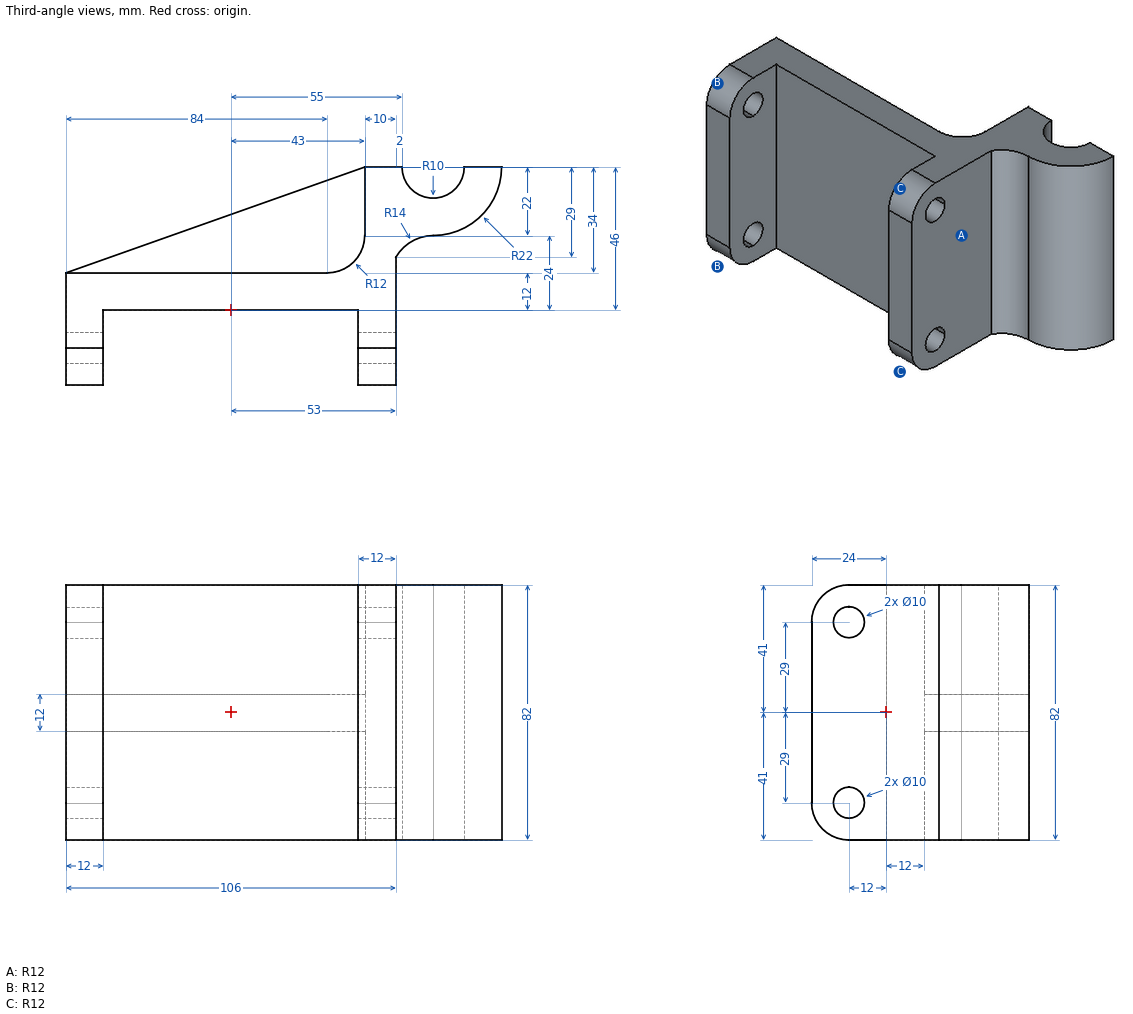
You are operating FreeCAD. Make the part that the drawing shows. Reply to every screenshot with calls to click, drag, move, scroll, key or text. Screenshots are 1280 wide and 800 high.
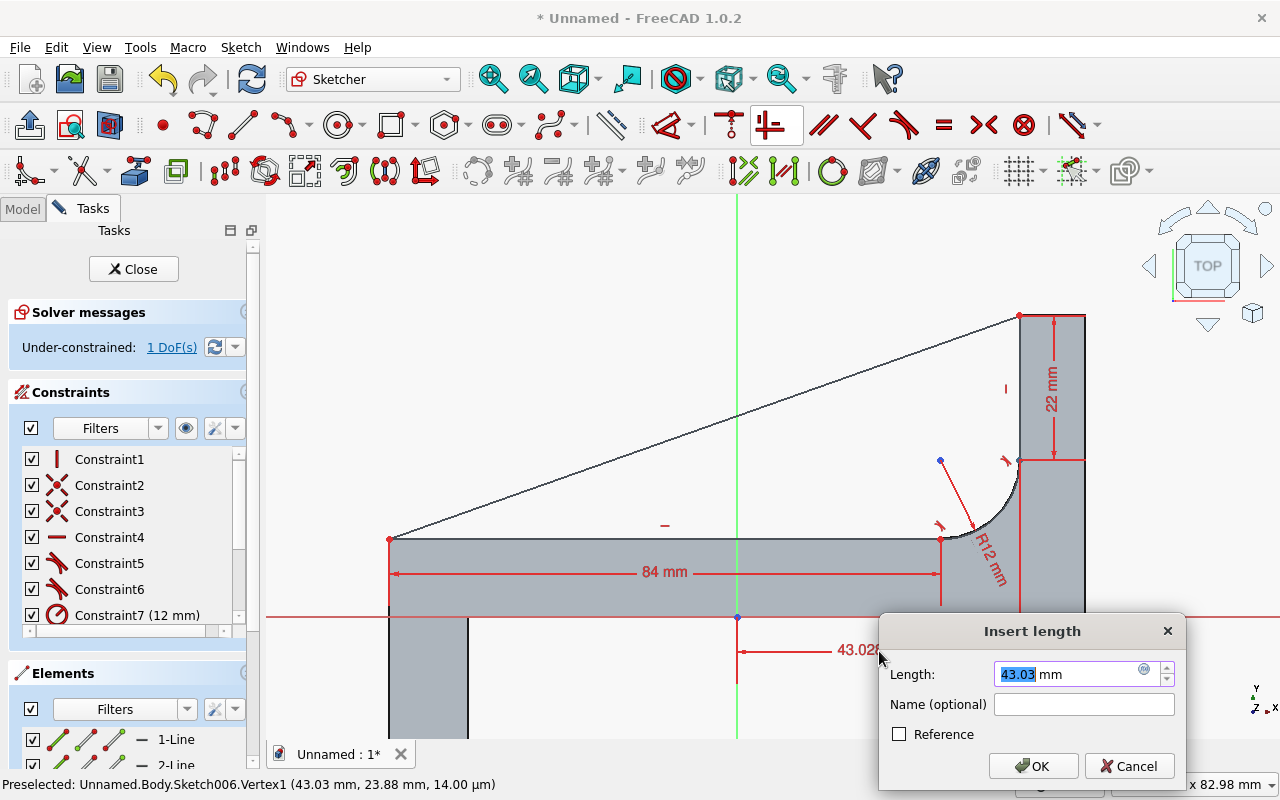
text(43)
key(Return)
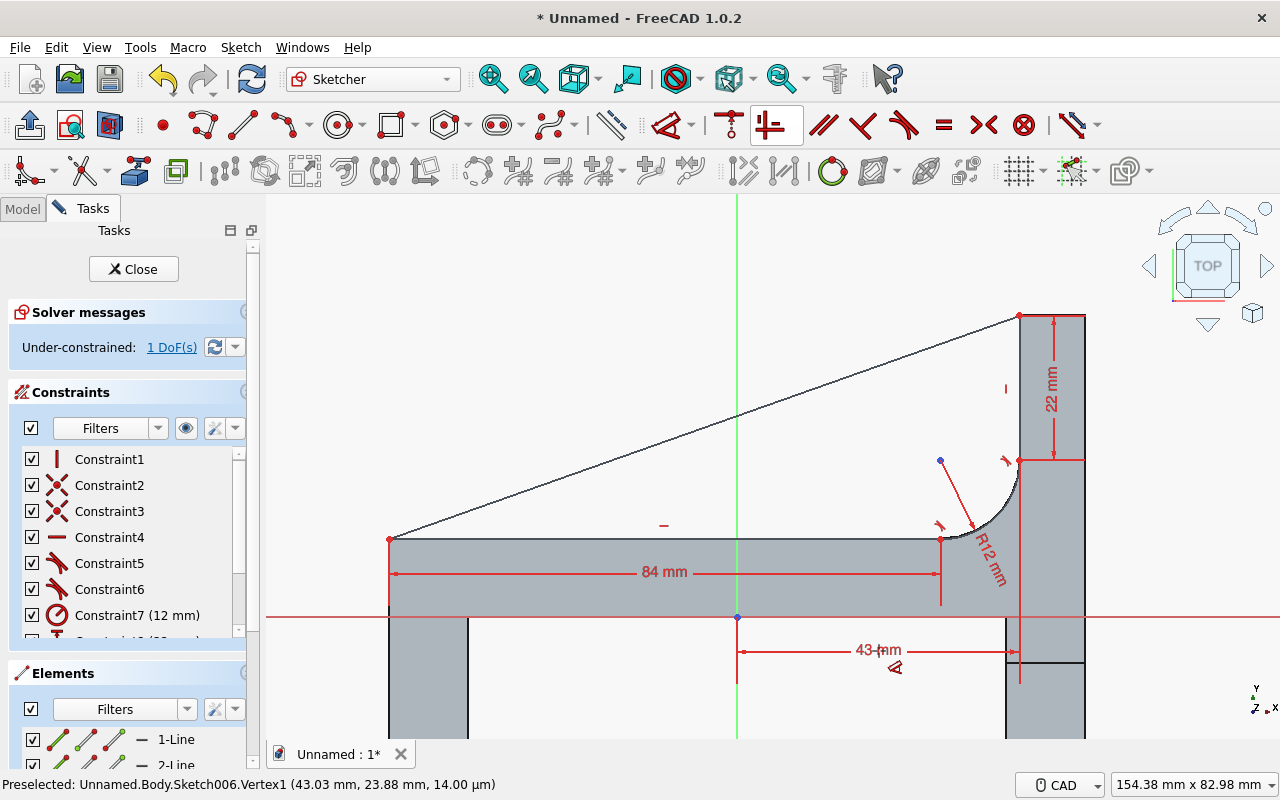
click(1020, 460)
click(1054, 539)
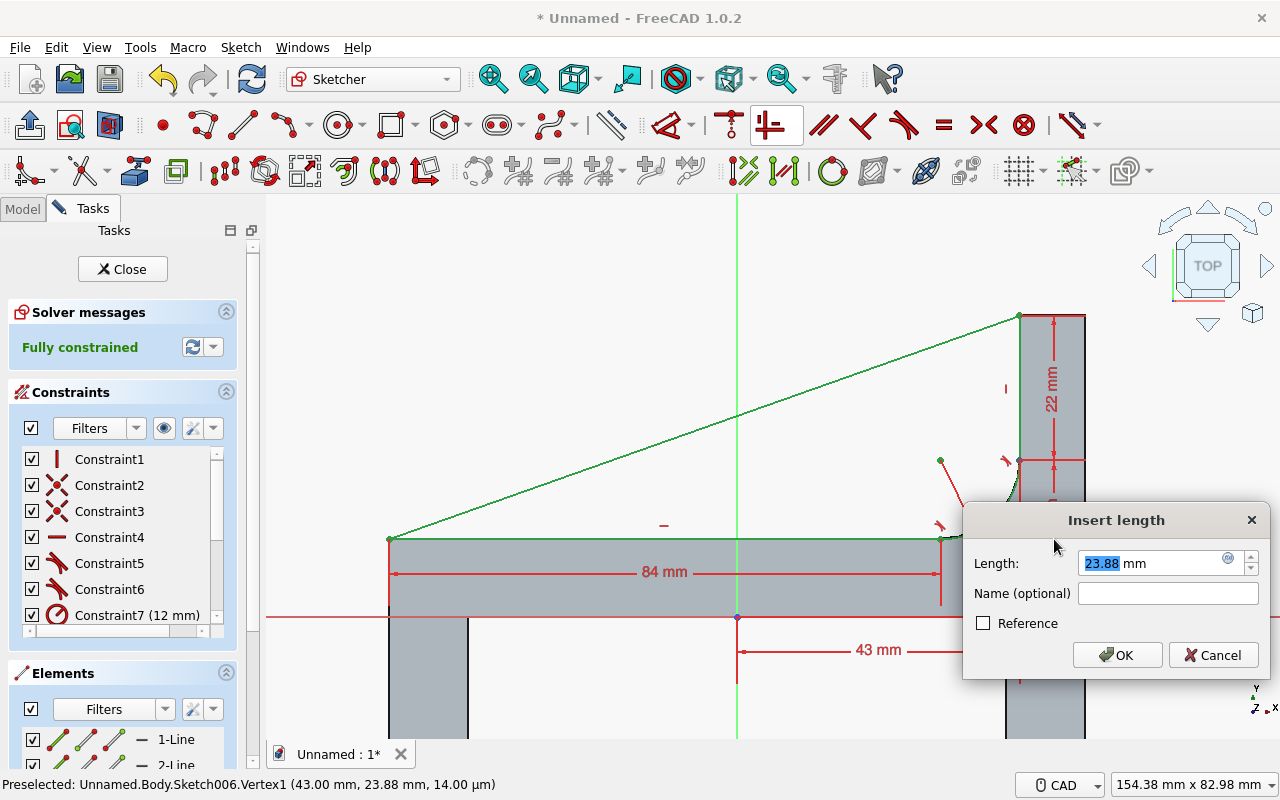
text(24)
key(Return)
key(Escape)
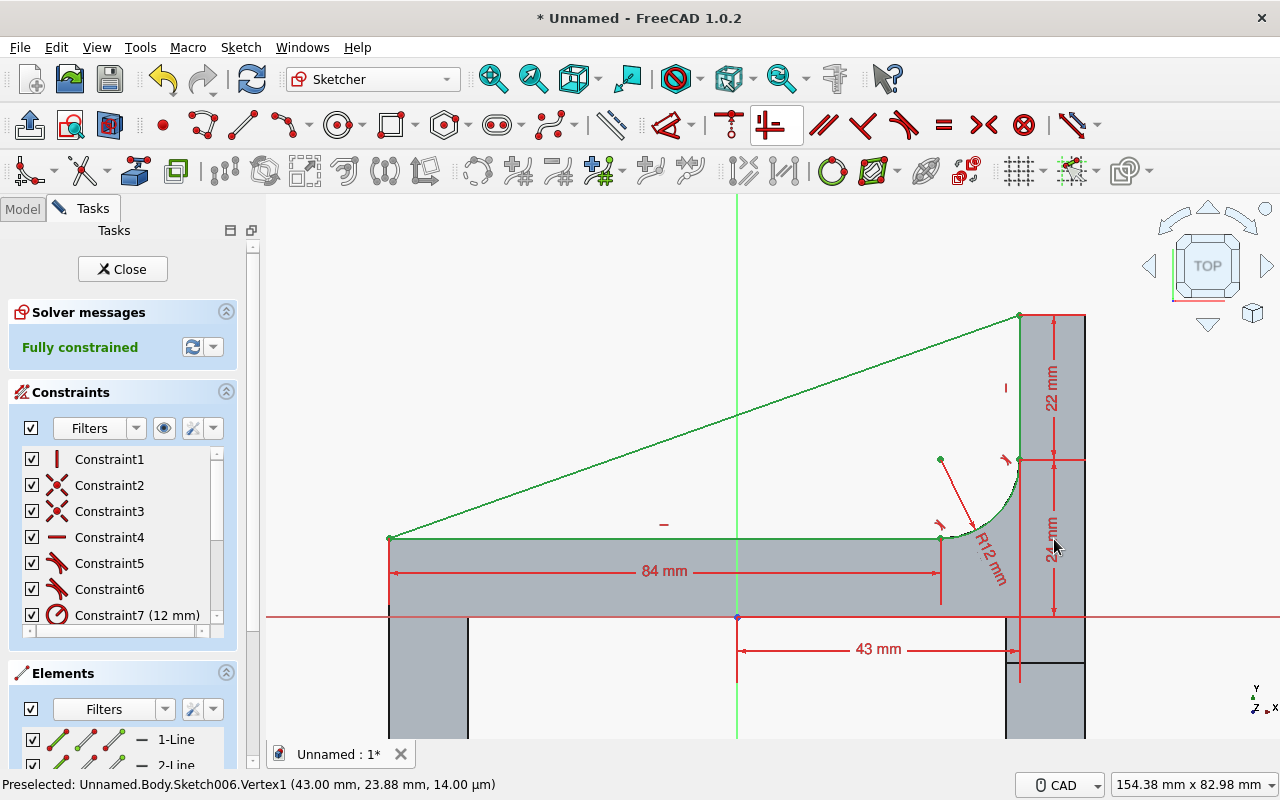
click(123, 269)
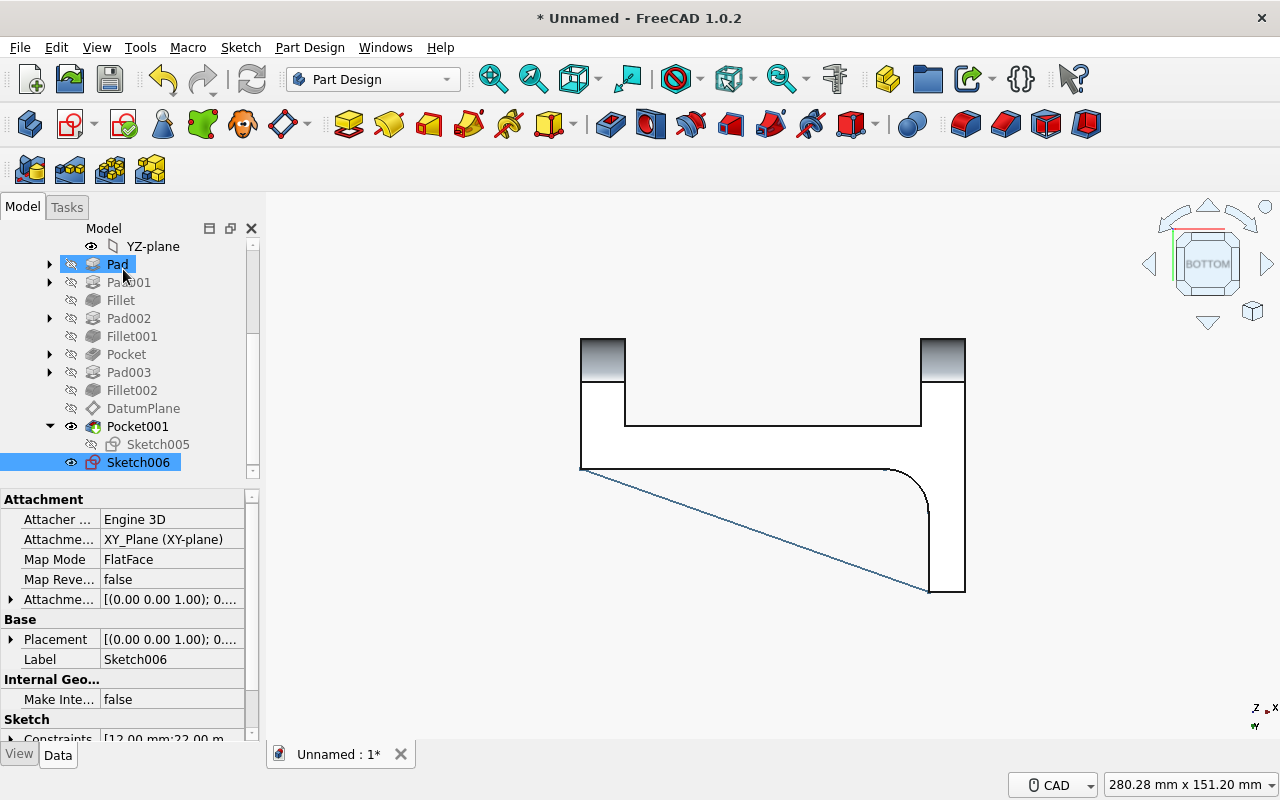
click(350, 124)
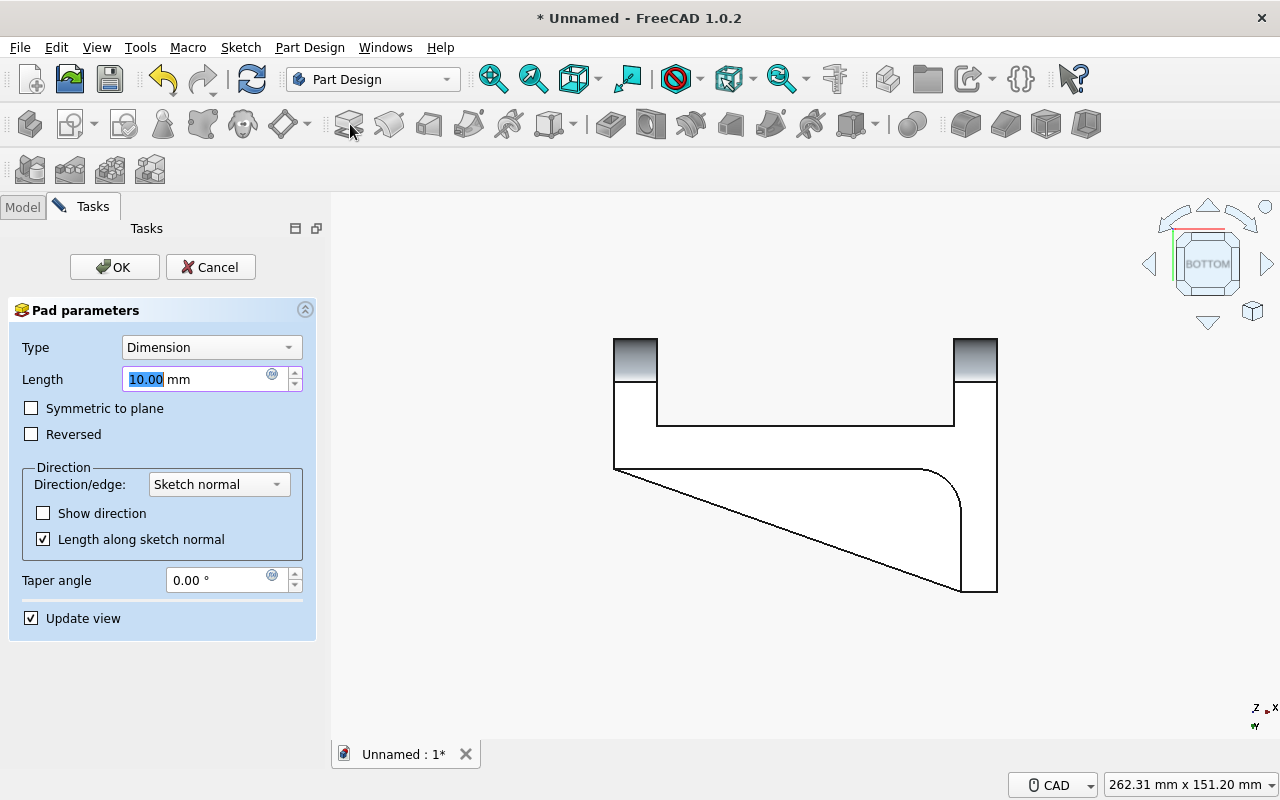
text(12)
key(Tab)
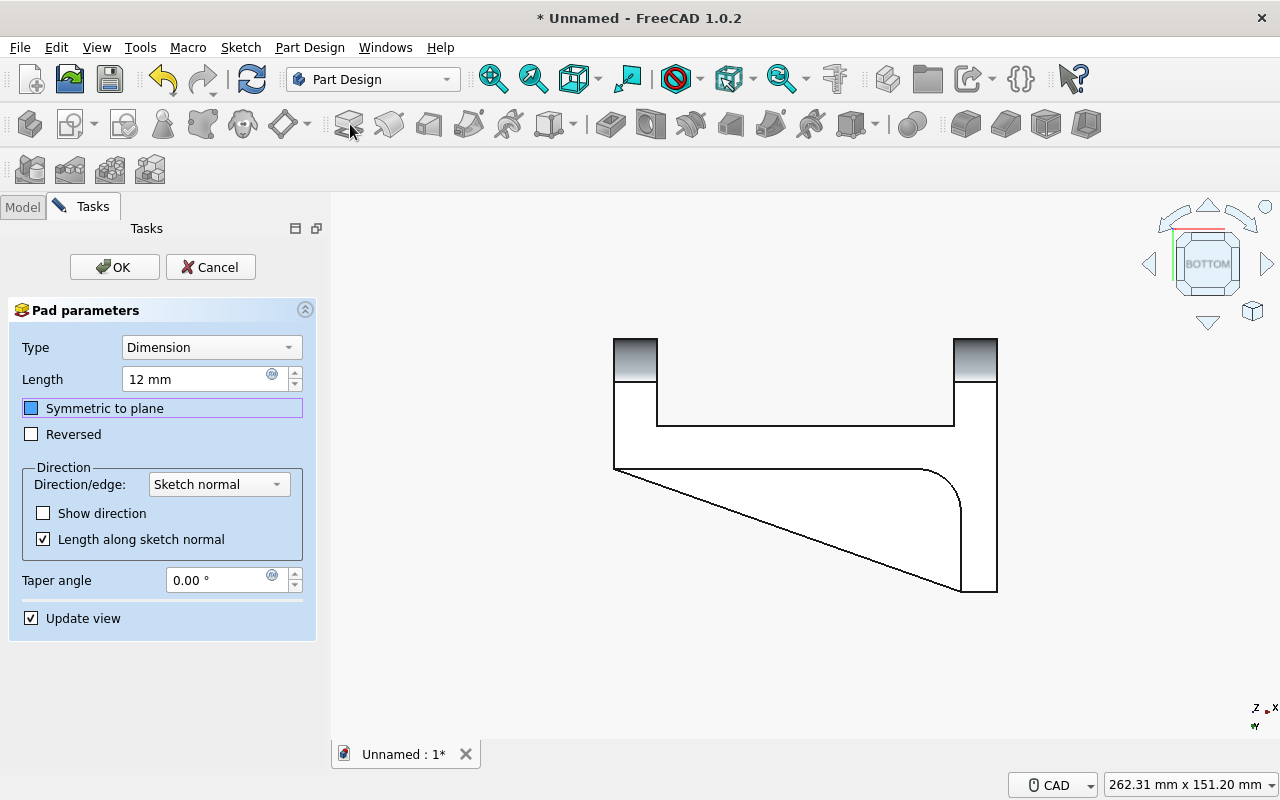
click(30, 408)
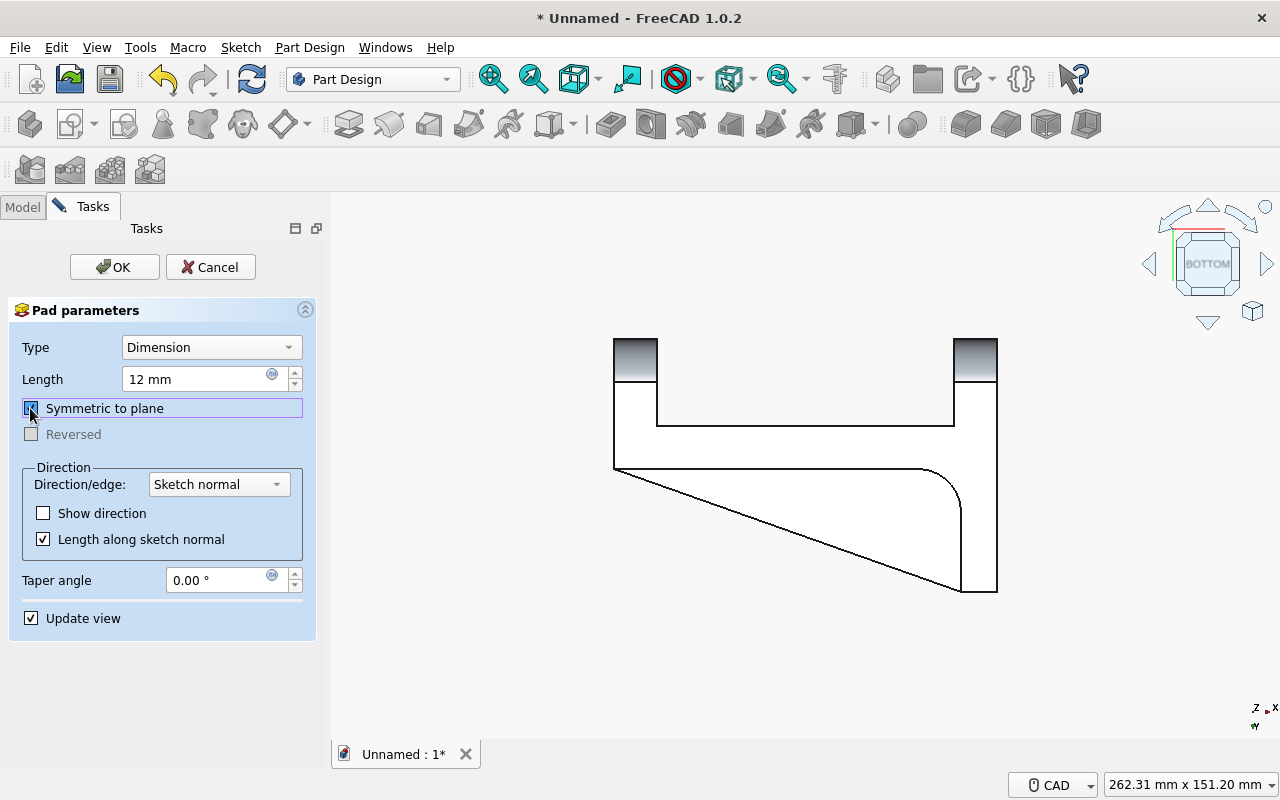
click(115, 267)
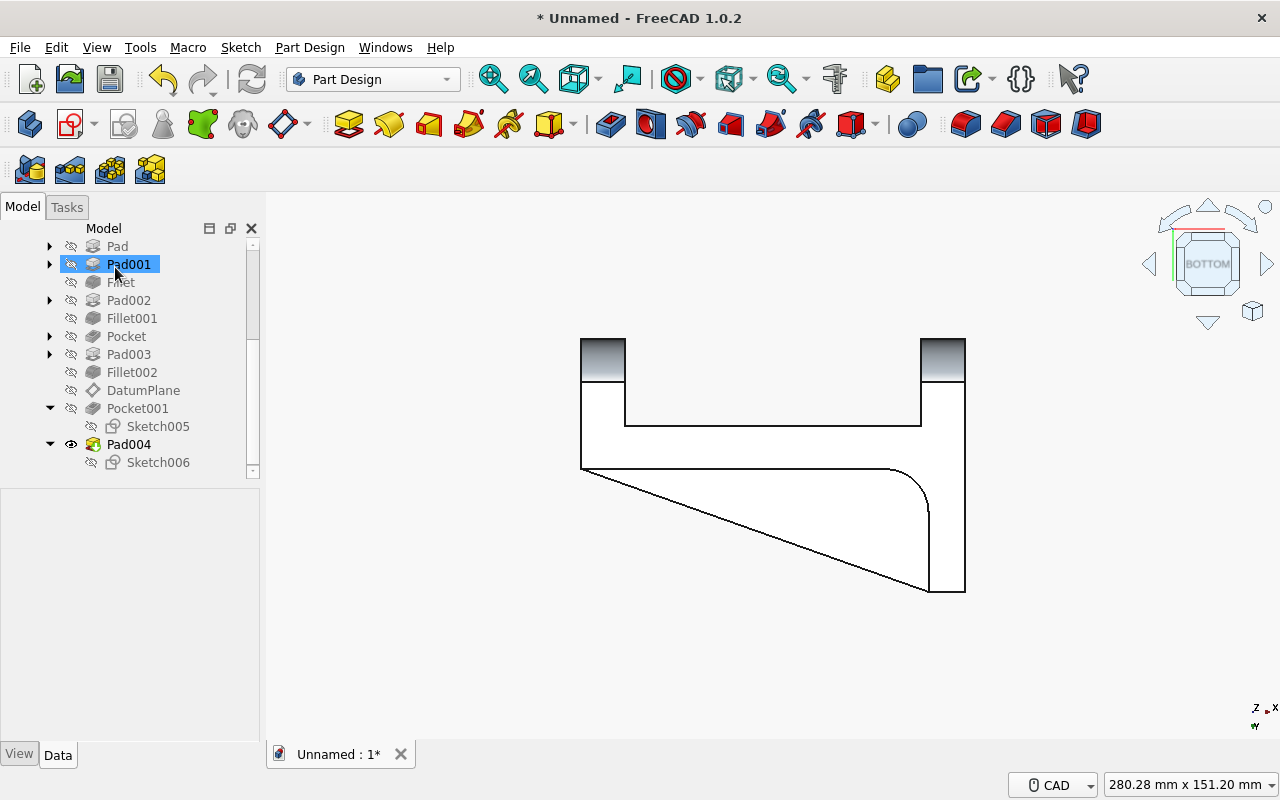
key(0)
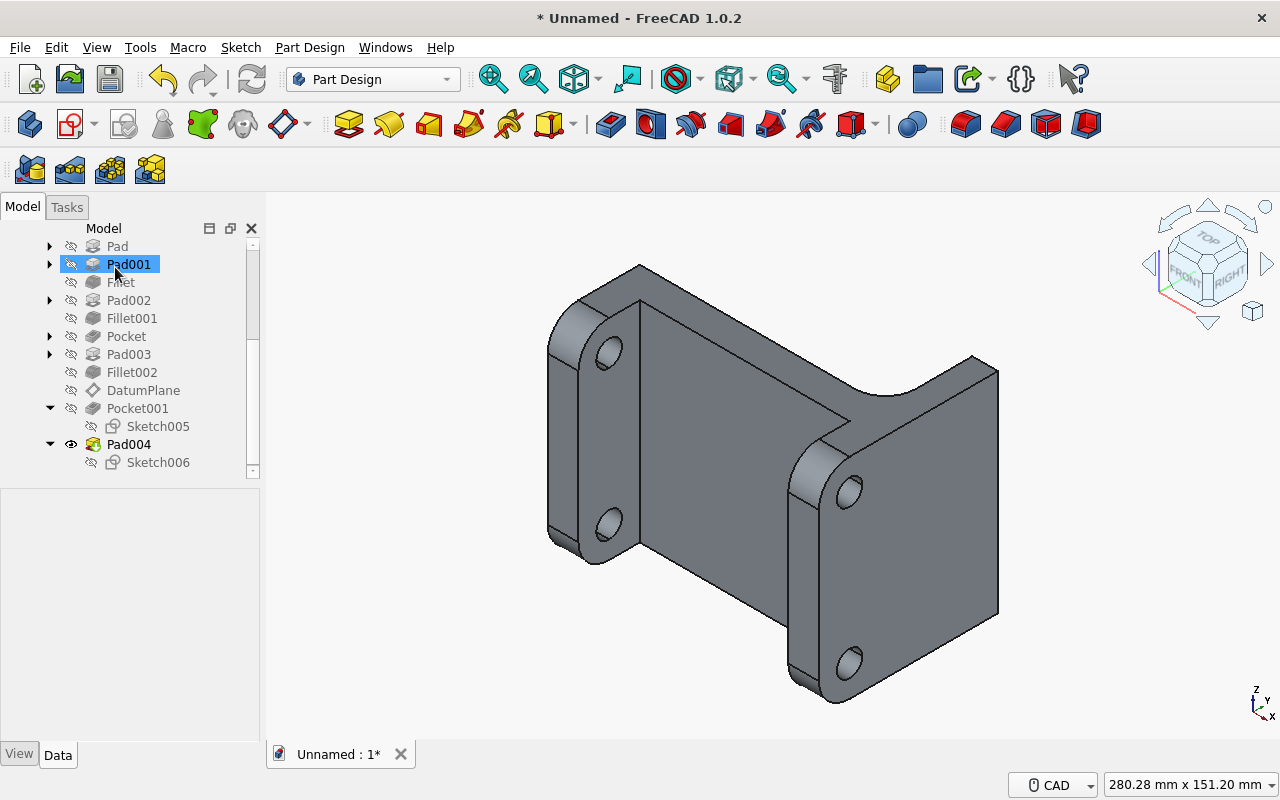
click(883, 414)